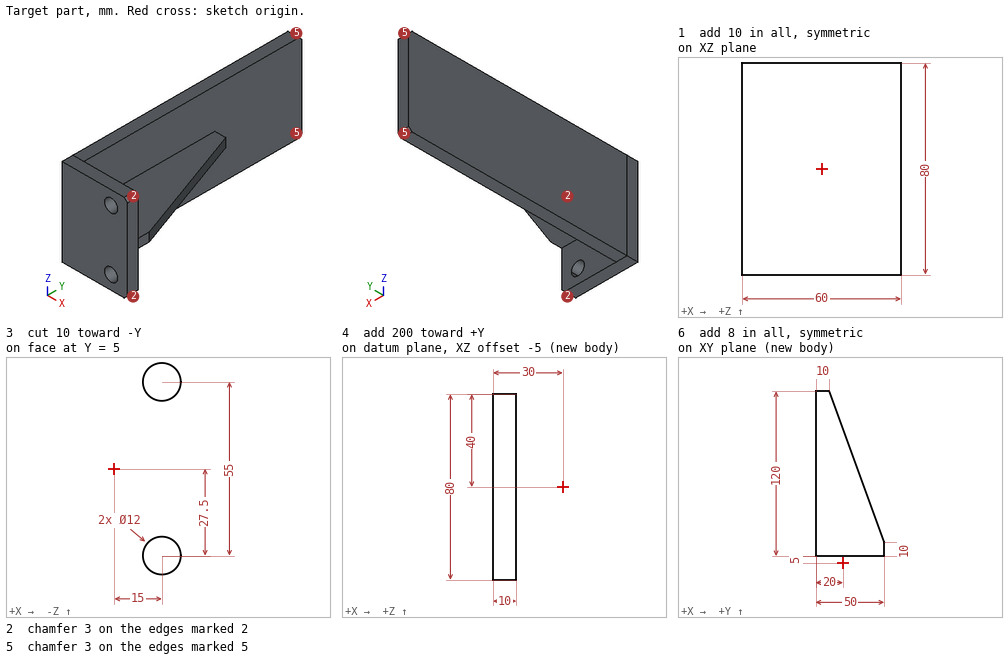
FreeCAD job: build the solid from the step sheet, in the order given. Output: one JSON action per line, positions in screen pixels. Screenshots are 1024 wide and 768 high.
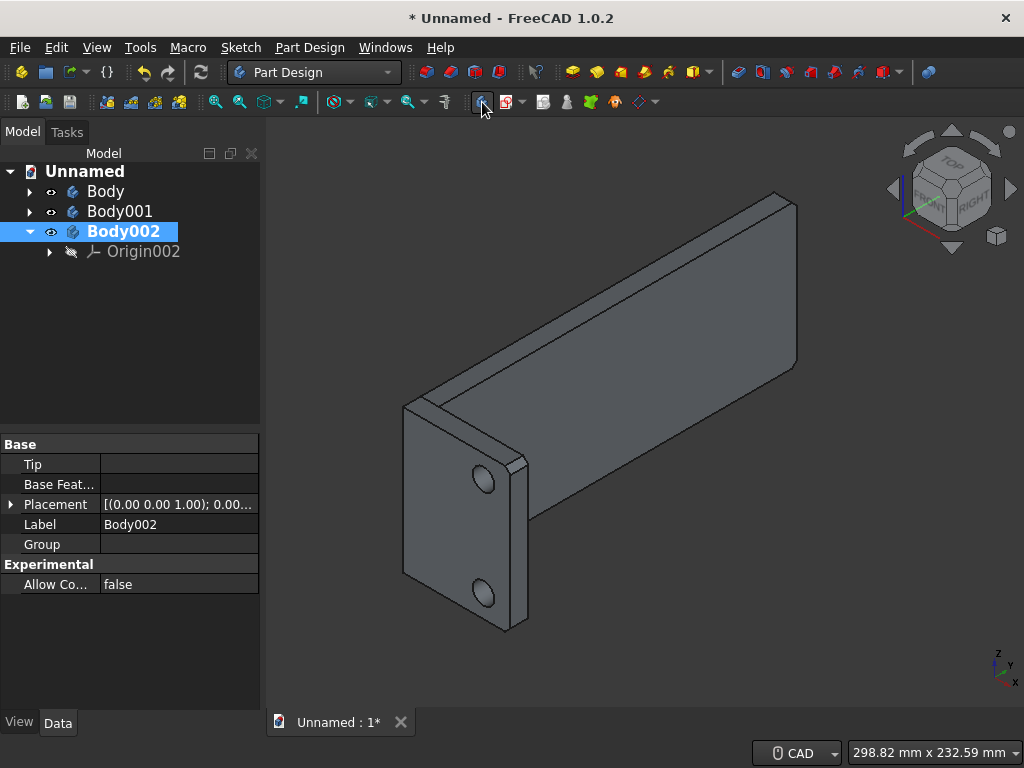
{"action": "left_click", "coordinate": [306, 667]}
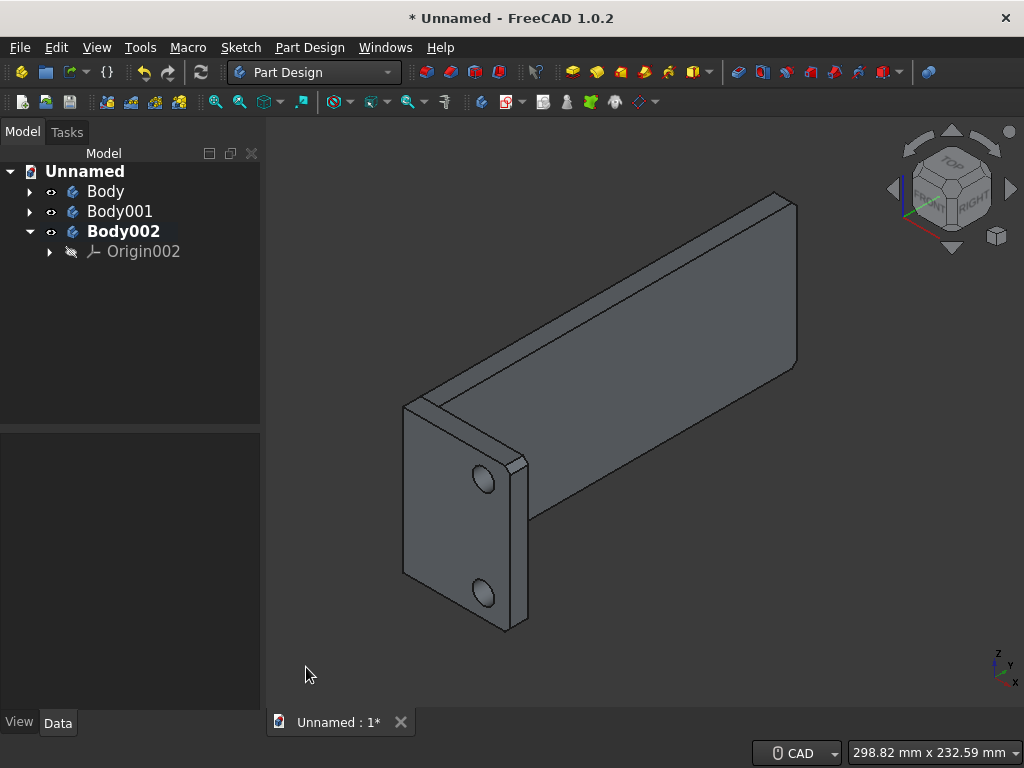
{"action": "left_click", "coordinate": [506, 102]}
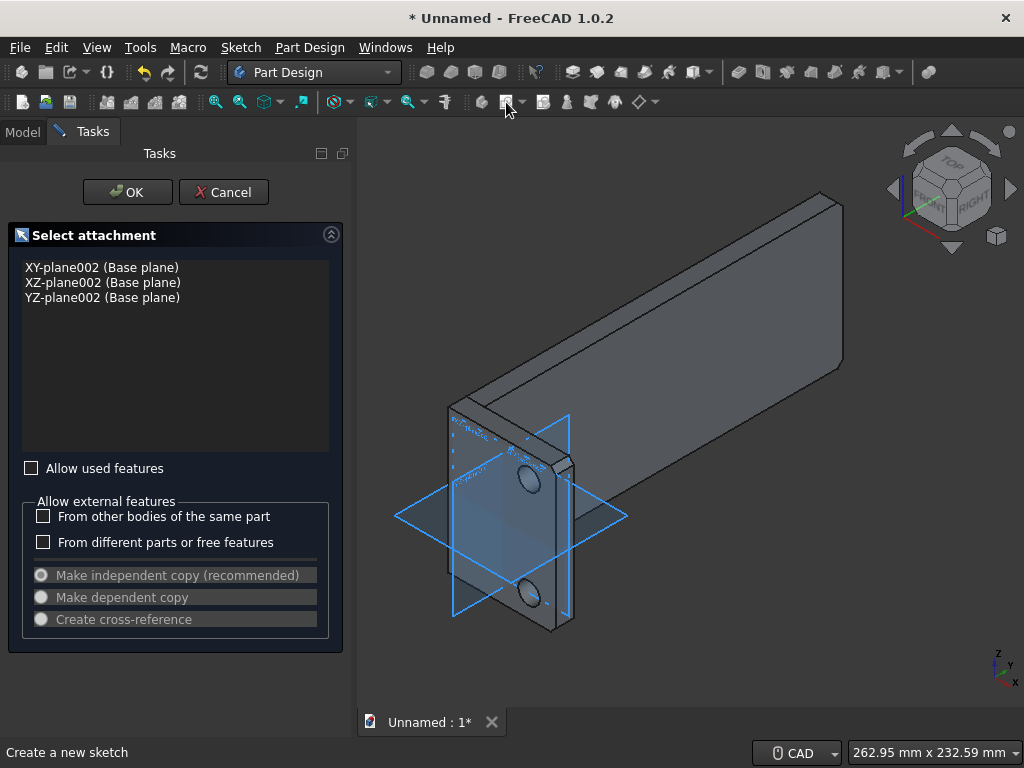
{"action": "left_click", "coordinate": [82, 268]}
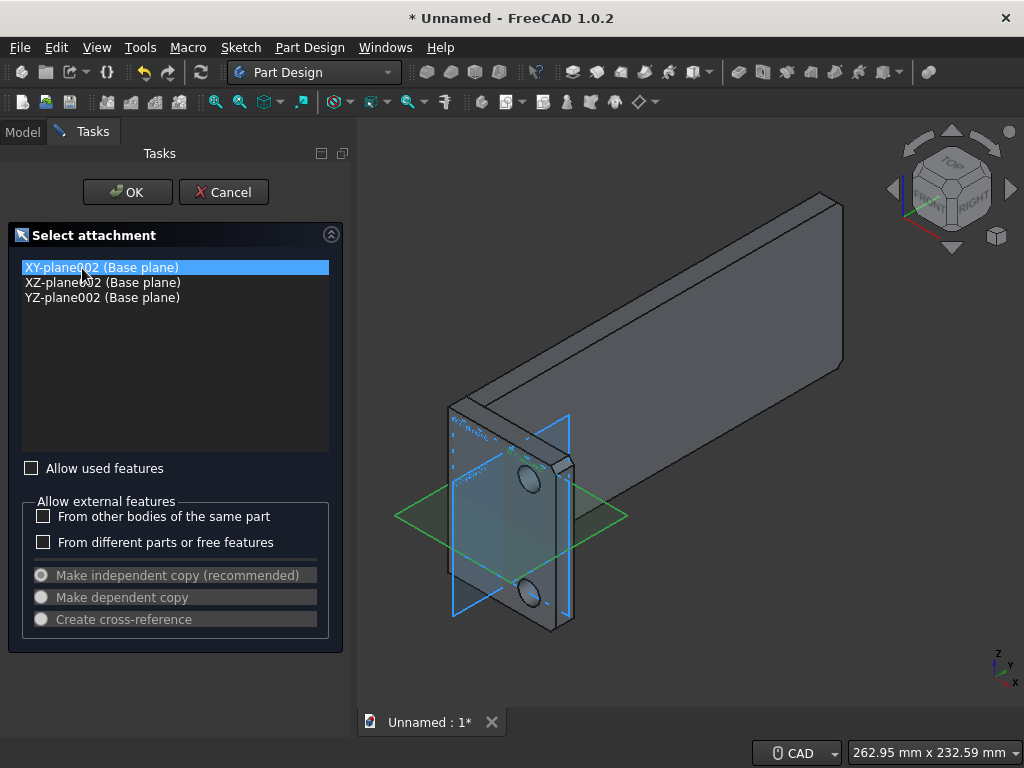
{"action": "left_click", "coordinate": [128, 192]}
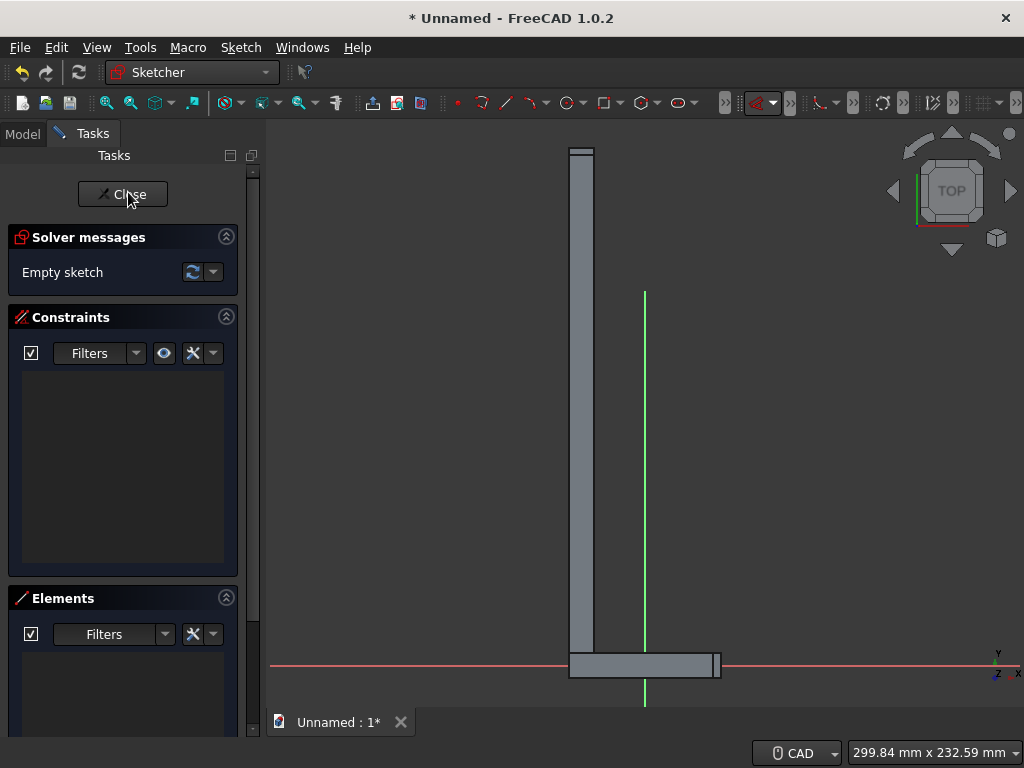
{"action": "scroll", "coordinate": [294, 147], "scroll_direction": "down", "scroll_amount": 1}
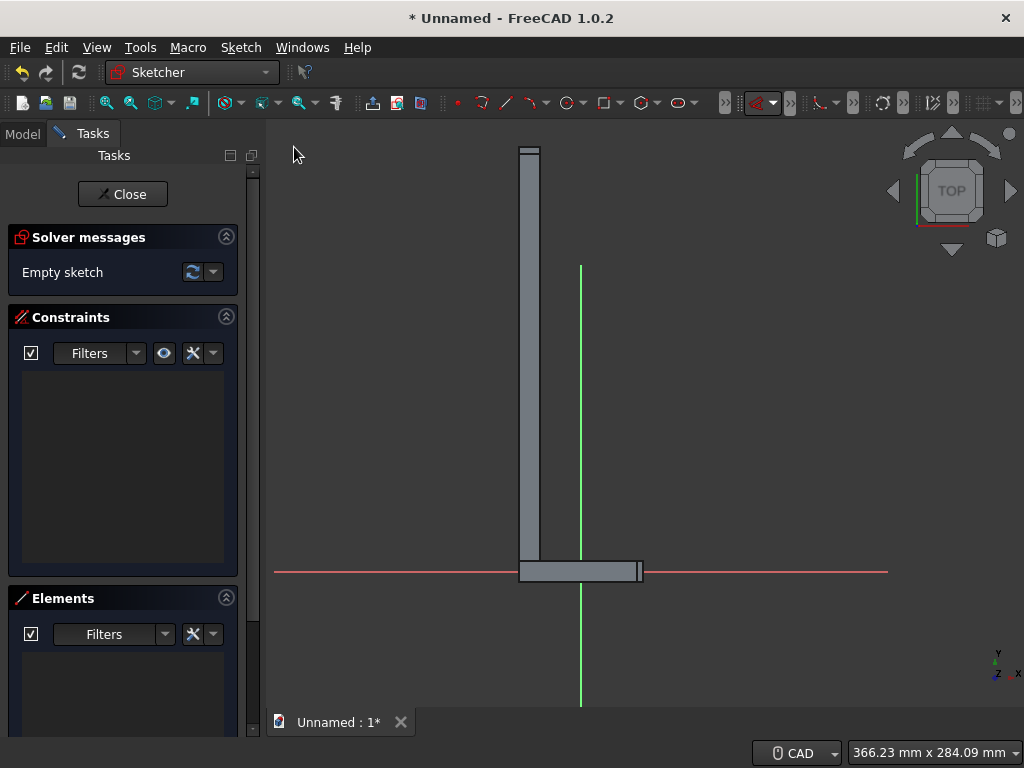
{"action": "scroll", "coordinate": [623, 502], "scroll_direction": "up", "scroll_amount": 2}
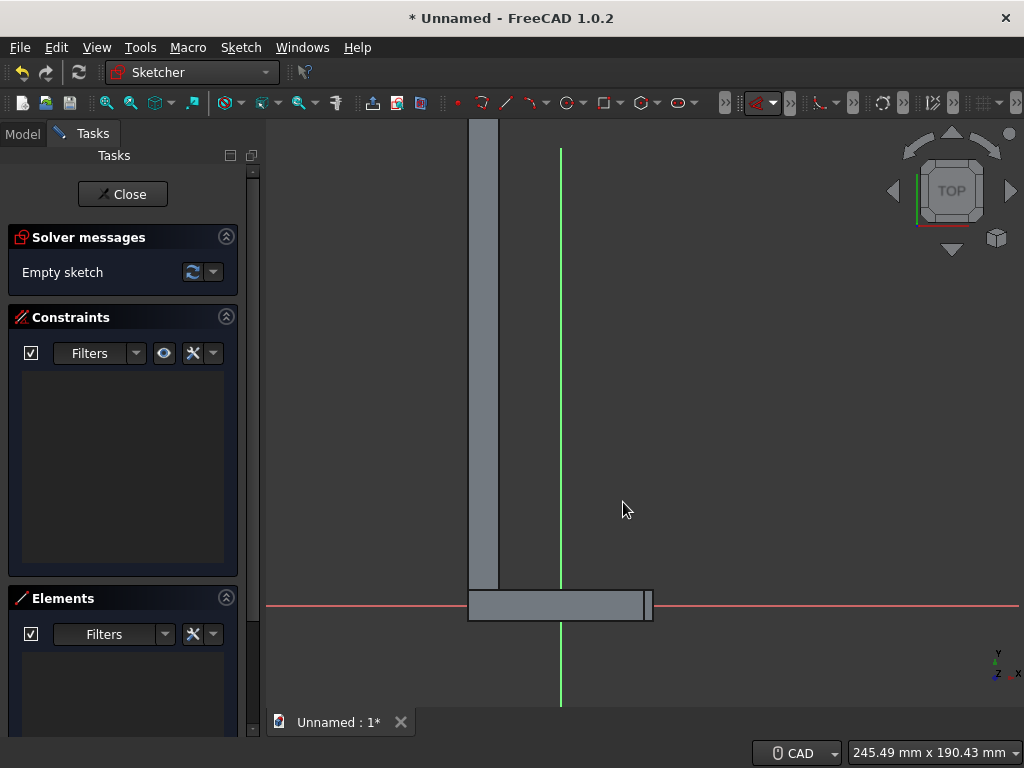
{"action": "left_click", "coordinate": [482, 104]}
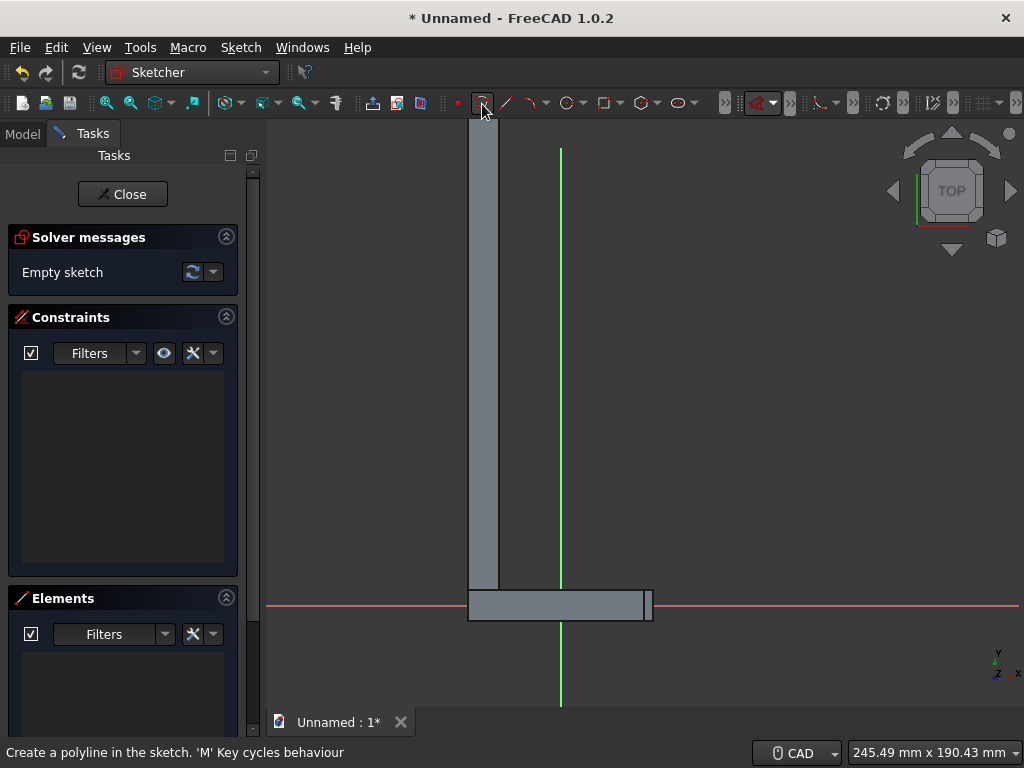
{"action": "left_click", "coordinate": [499, 590]}
{"action": "left_click", "coordinate": [653, 590]}
{"action": "left_click", "coordinate": [653, 559]}
{"action": "left_click", "coordinate": [530, 220]}
{"action": "left_click", "coordinate": [499, 220]}
{"action": "left_click", "coordinate": [499, 591]}
{"action": "key", "text": "Escape"}
{"action": "key", "text": "Escape"}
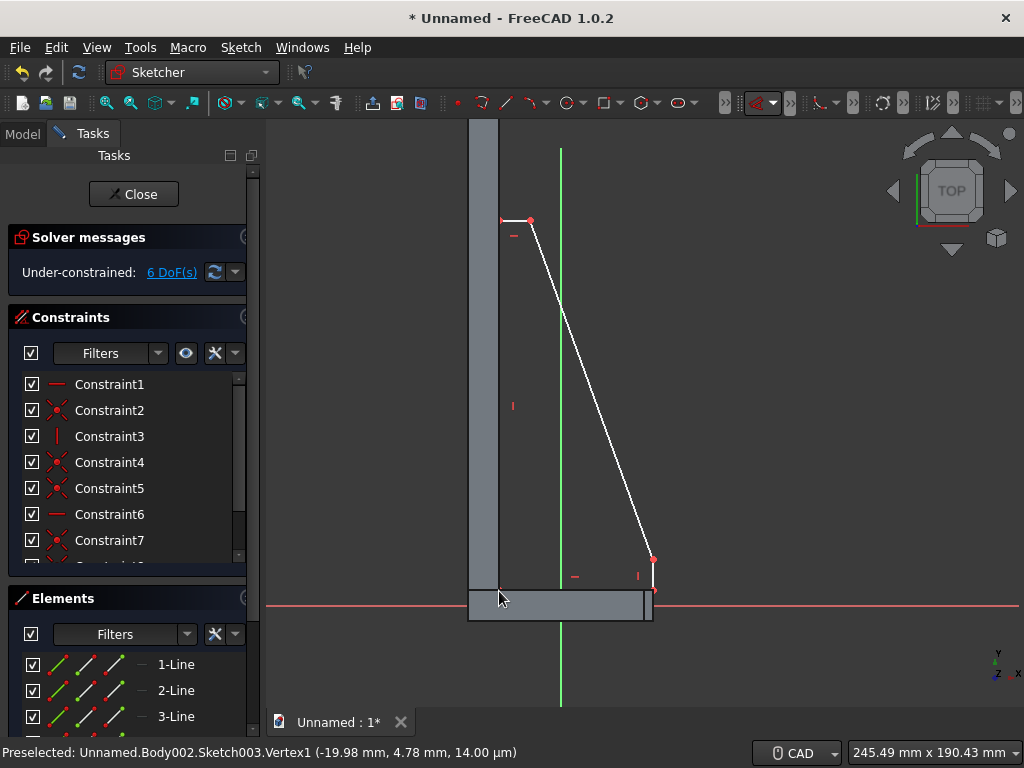
{"action": "left_click", "coordinate": [545, 591]}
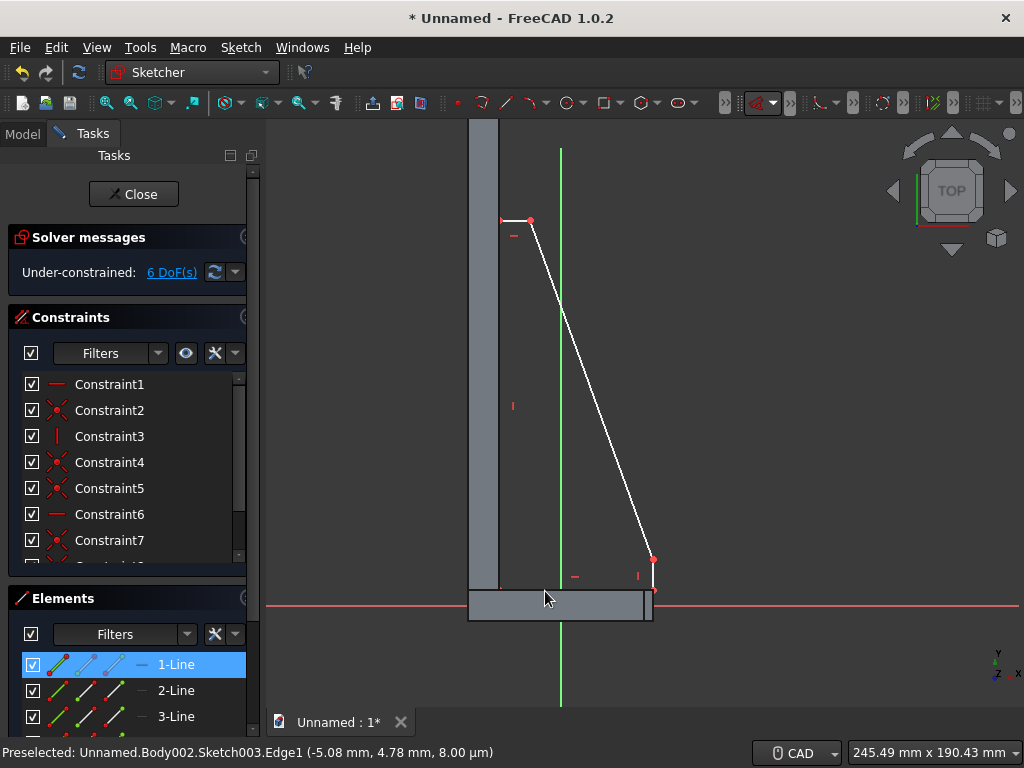
{"action": "left_click", "coordinate": [776, 104]}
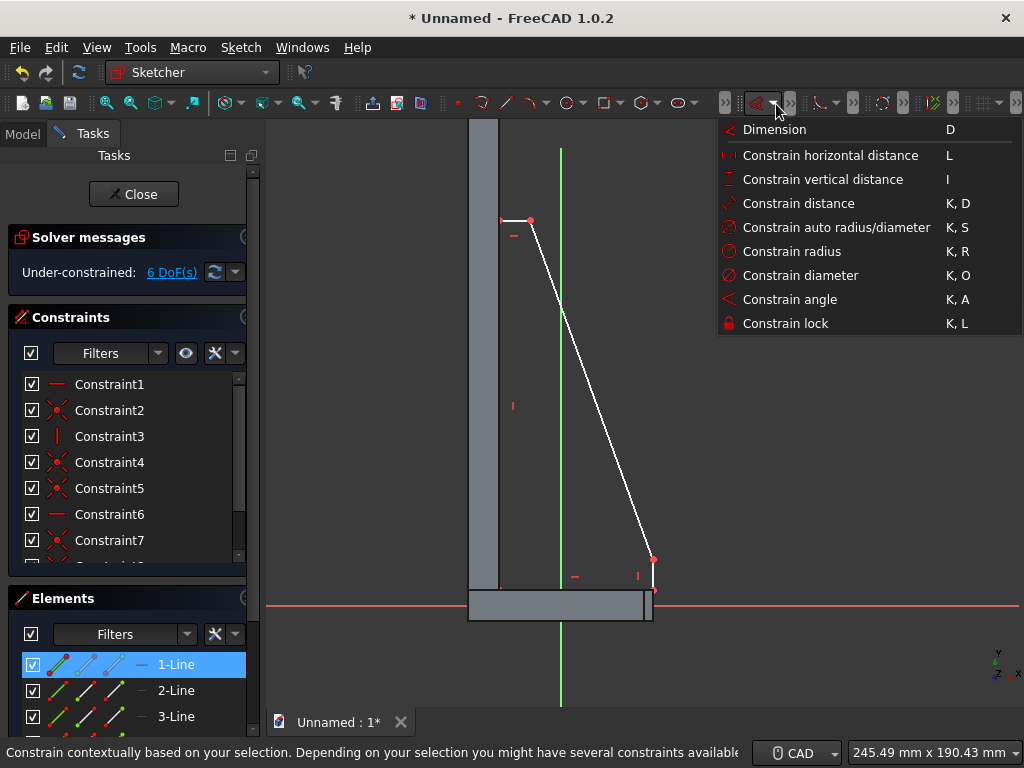
{"action": "left_click", "coordinate": [870, 155]}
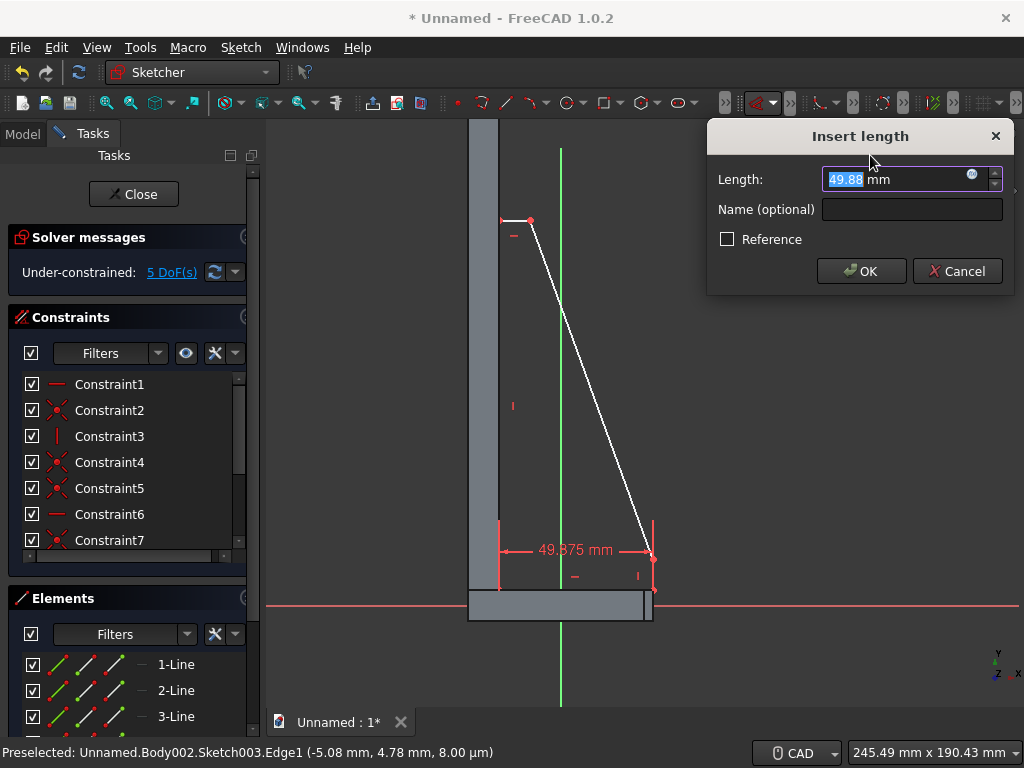
{"action": "type", "text": "50"}
{"action": "key", "text": "Return"}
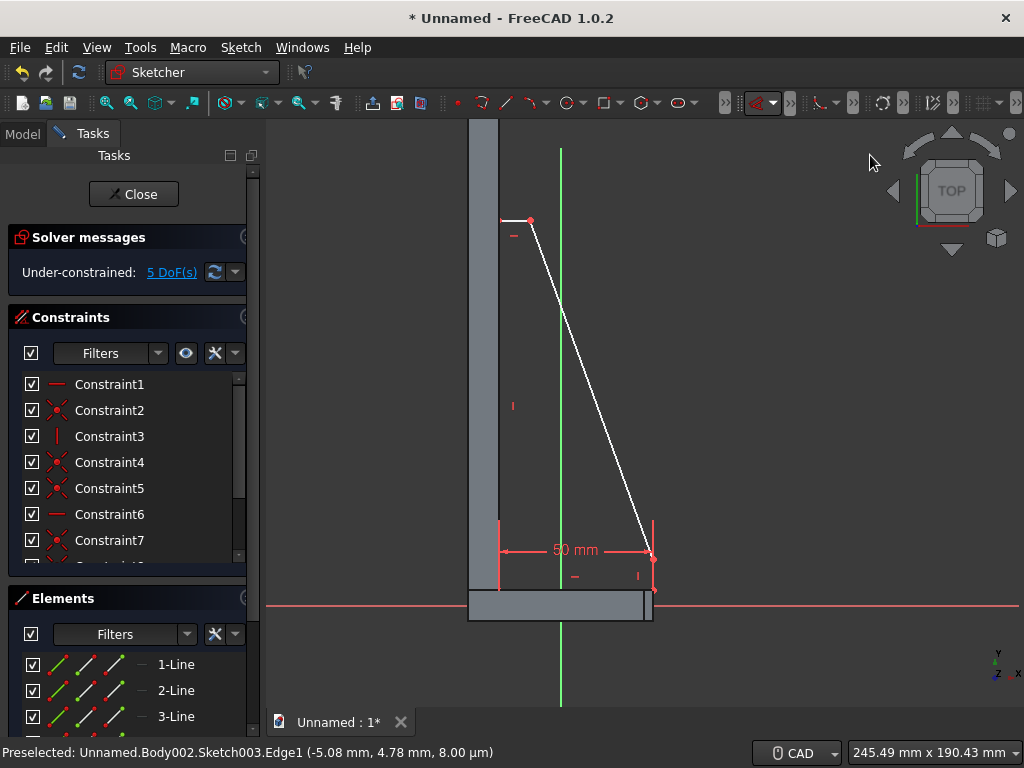
{"action": "scroll", "coordinate": [653, 582], "scroll_direction": "up", "scroll_amount": 2}